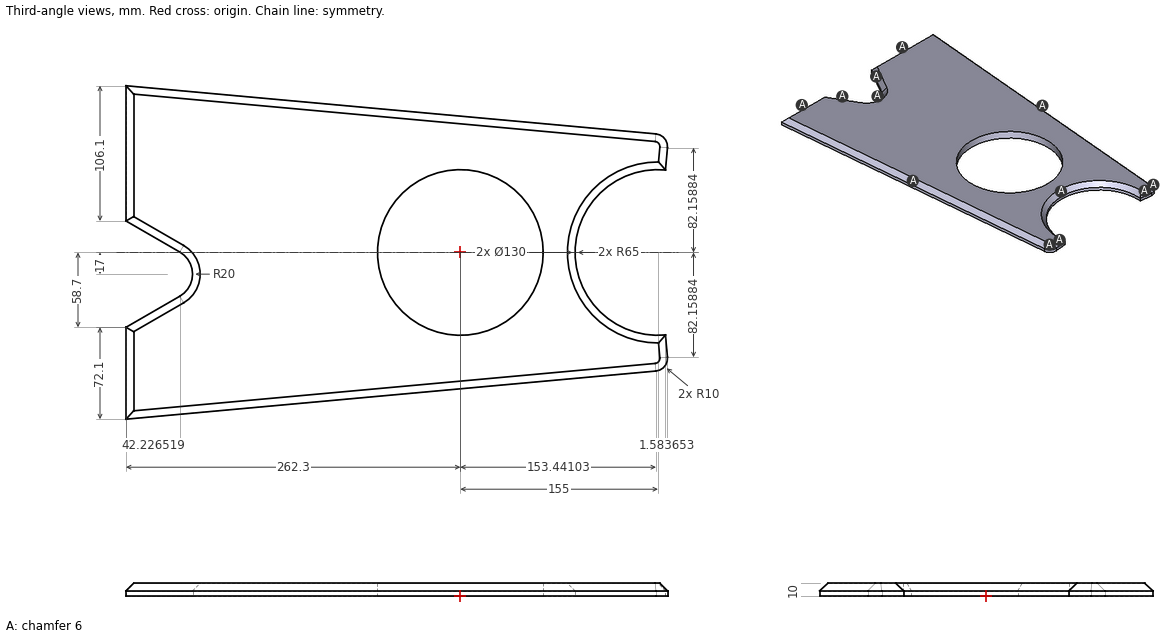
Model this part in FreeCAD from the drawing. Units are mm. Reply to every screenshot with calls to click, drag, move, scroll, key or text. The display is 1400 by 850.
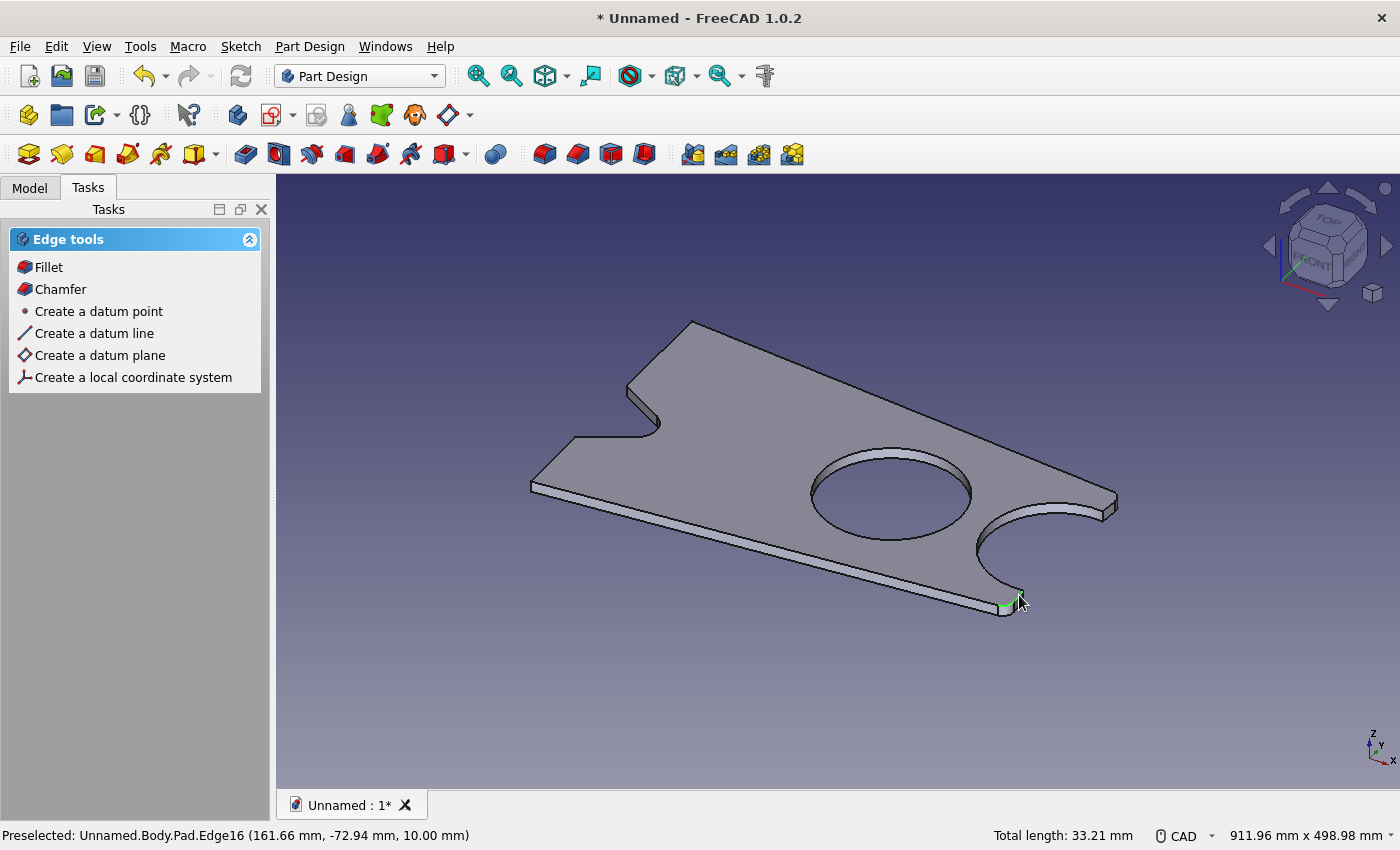
click(987, 525, ctrl)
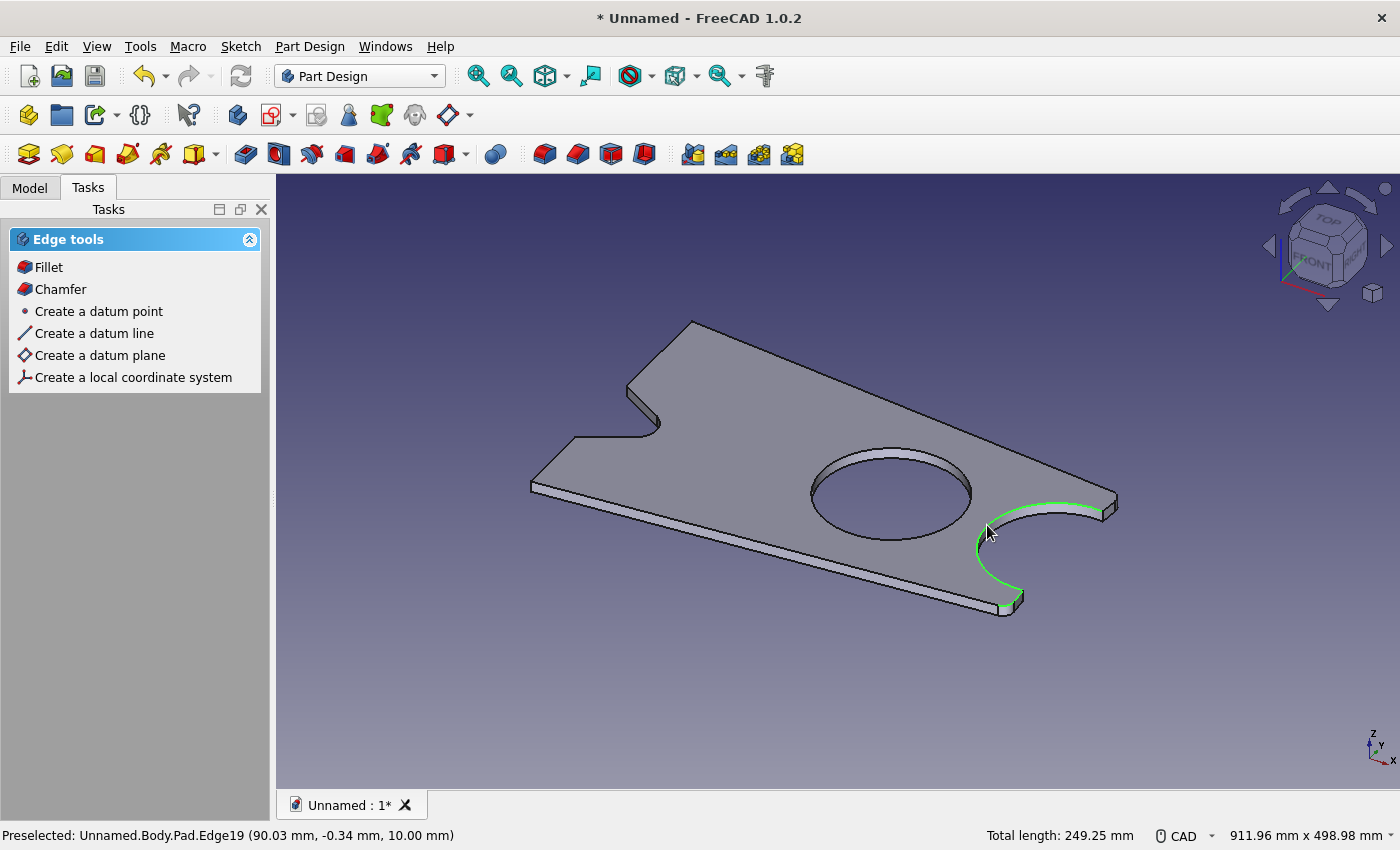
click(1109, 505, ctrl)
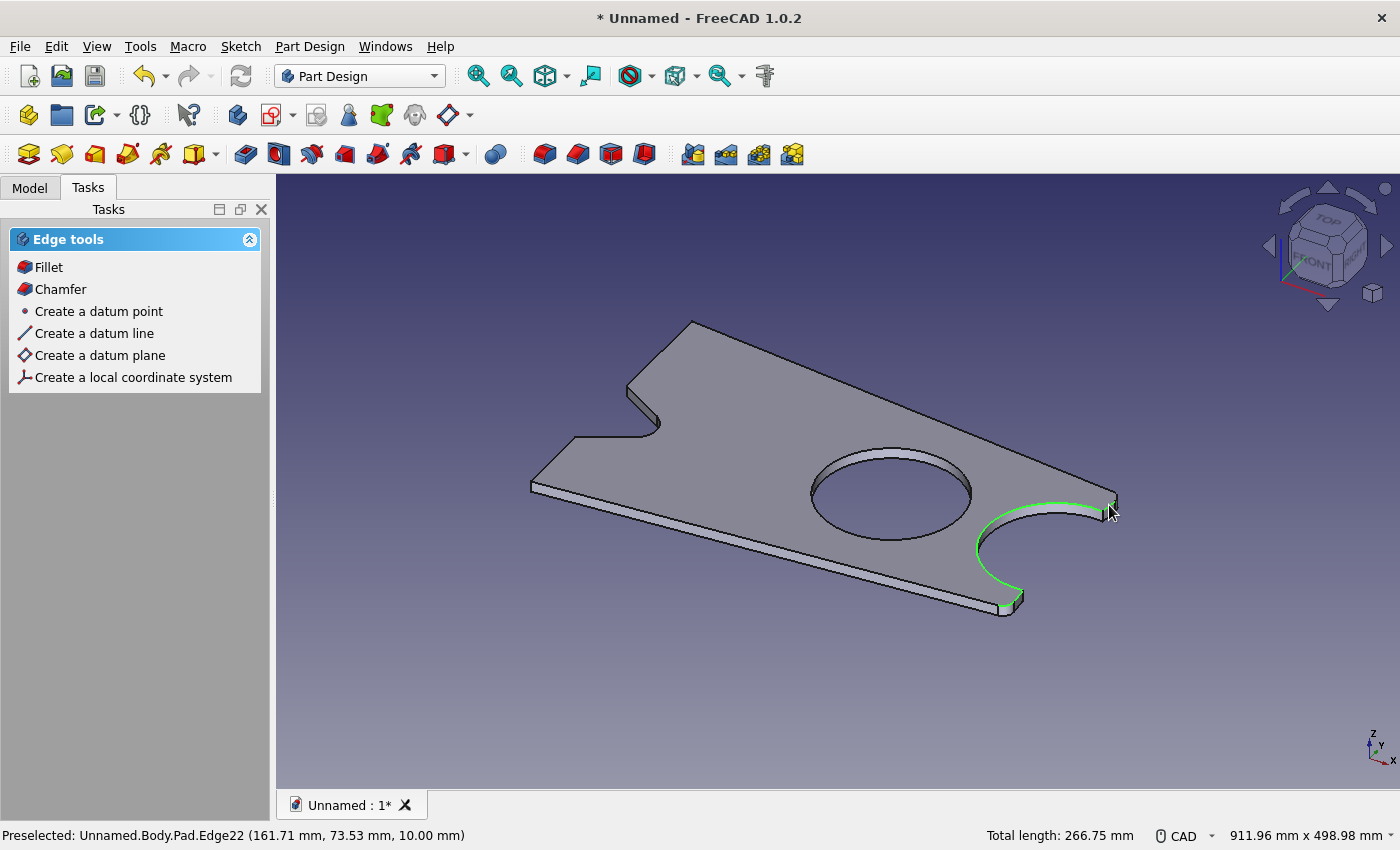
click(1117, 494, ctrl)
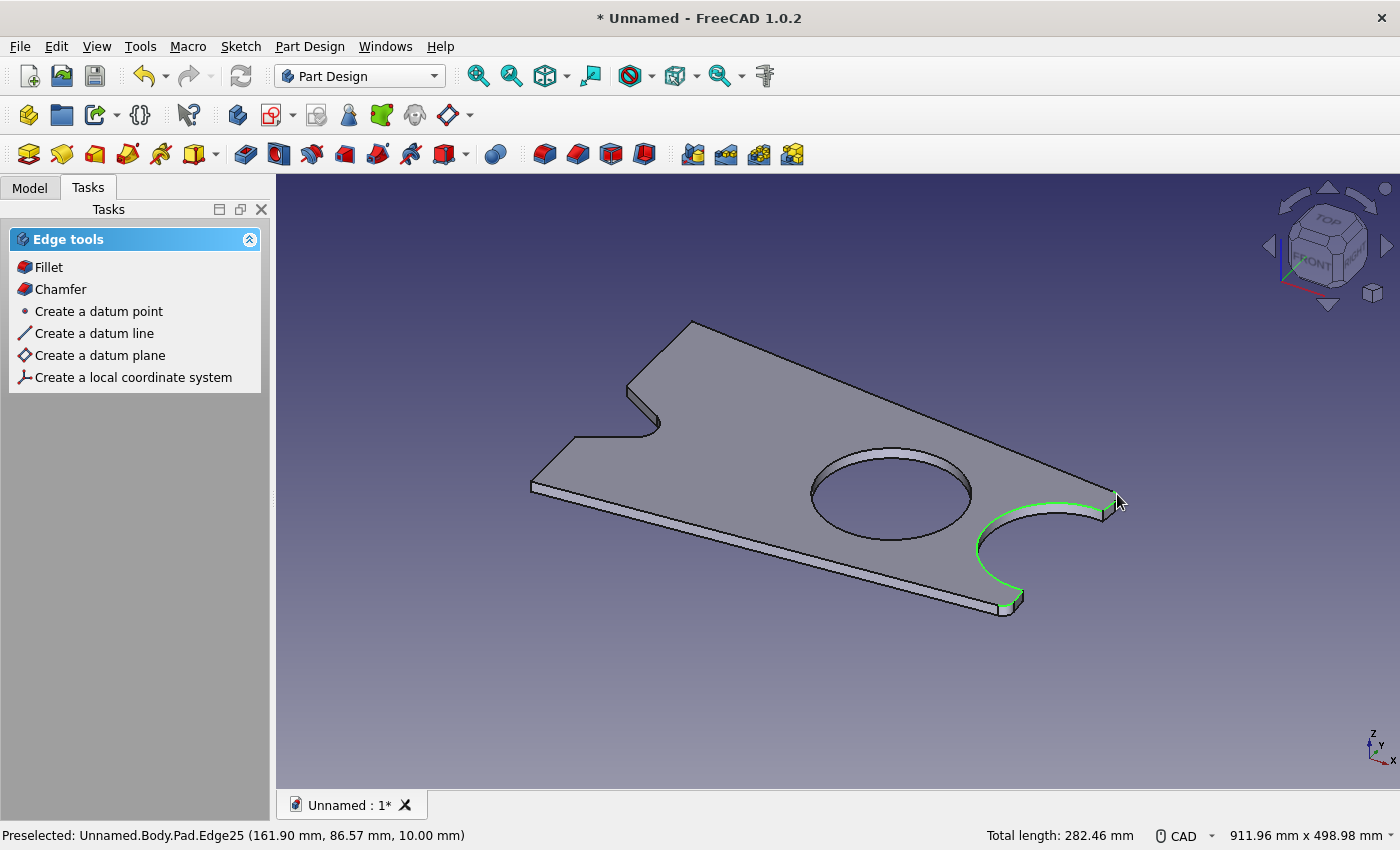
click(642, 400, ctrl)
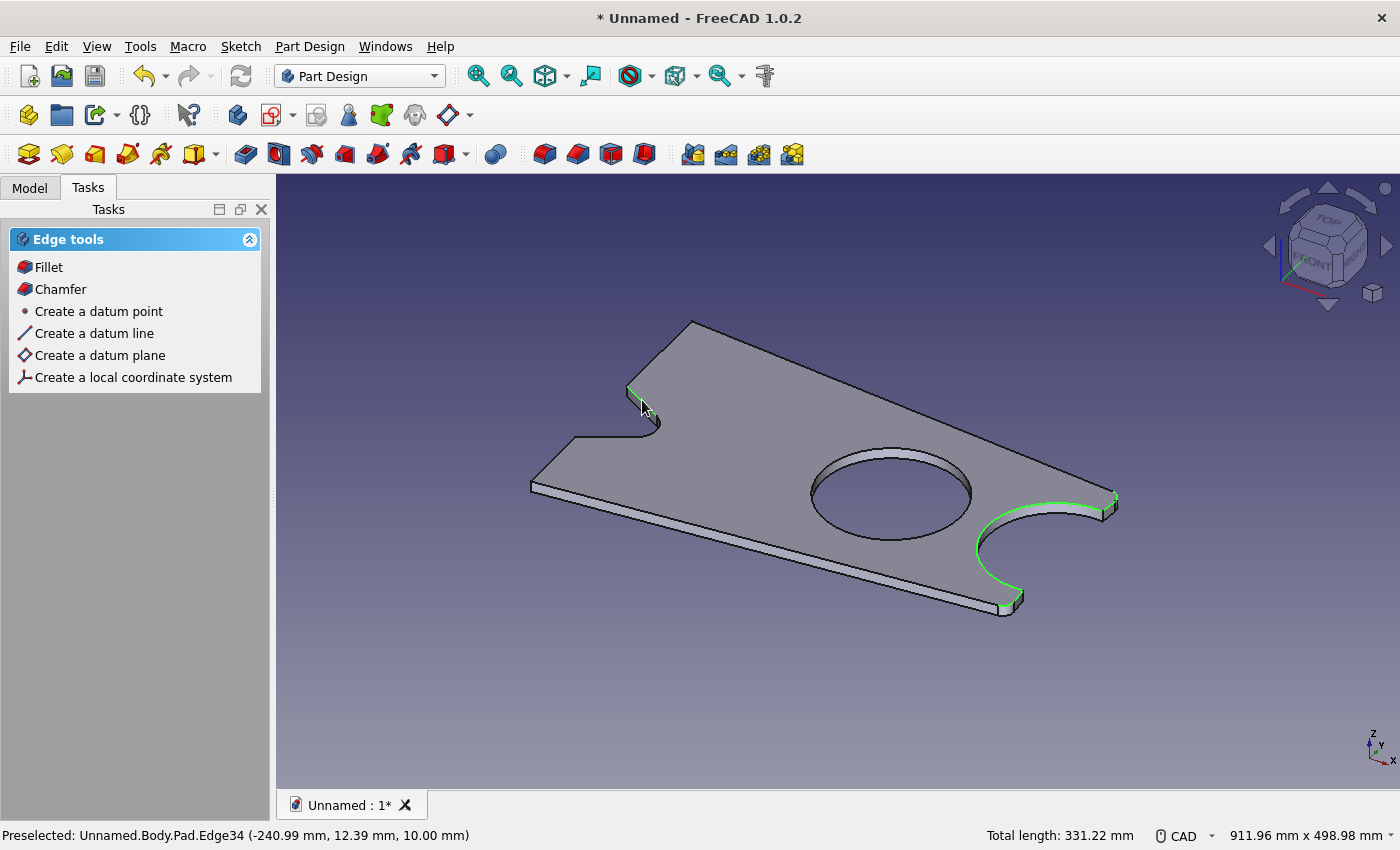
click(657, 429, ctrl)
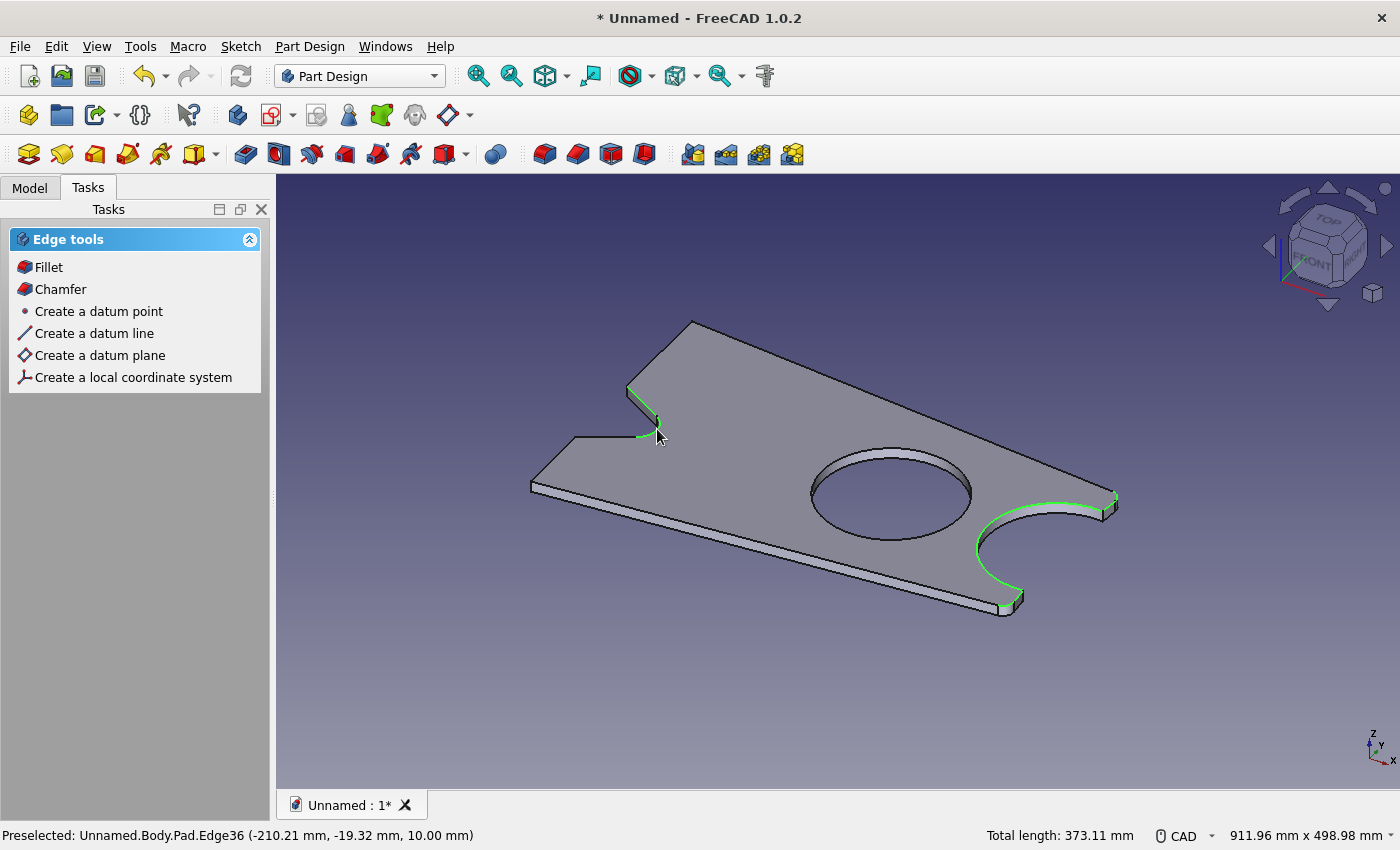
click(764, 542, ctrl)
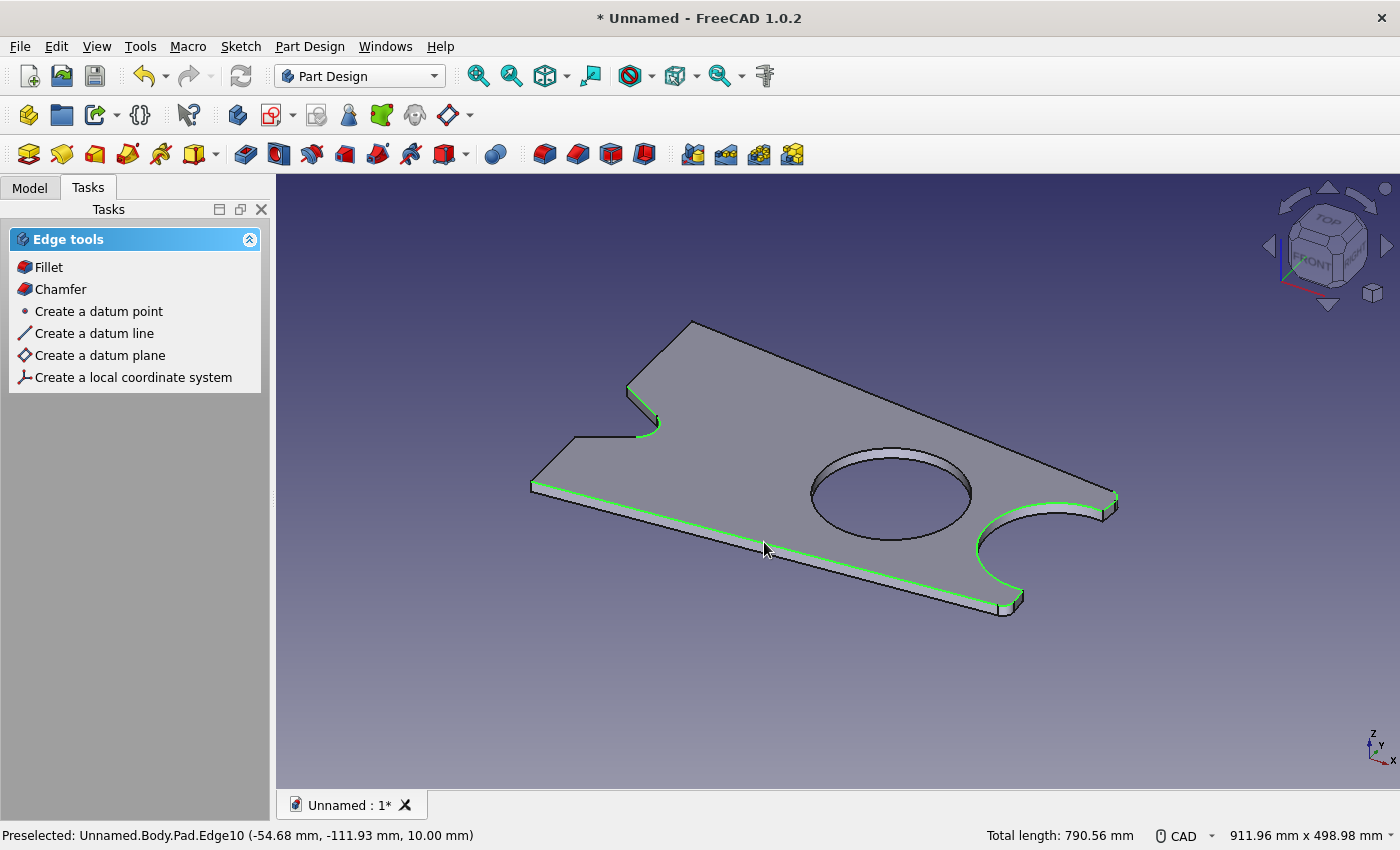
key(0)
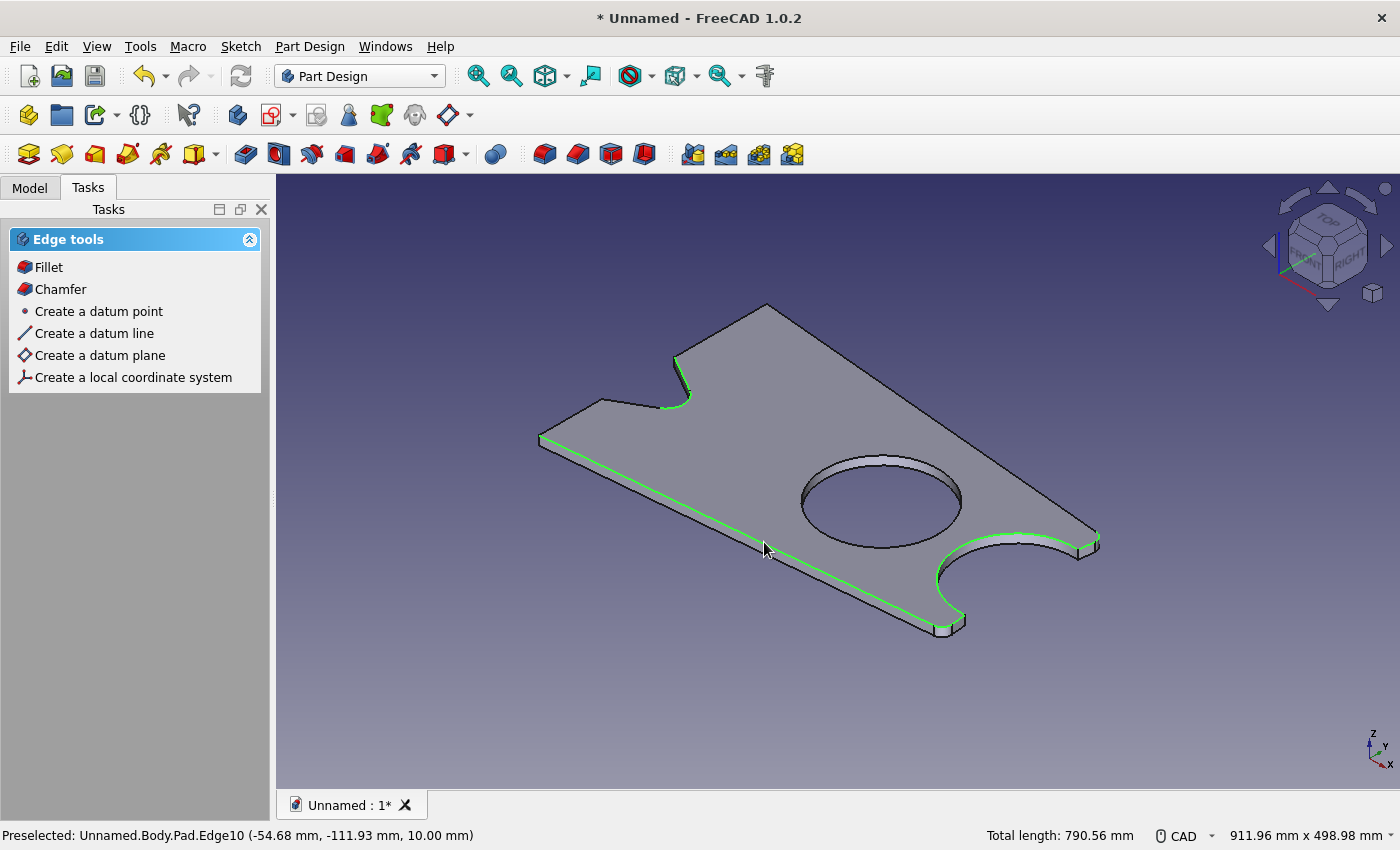
key(2)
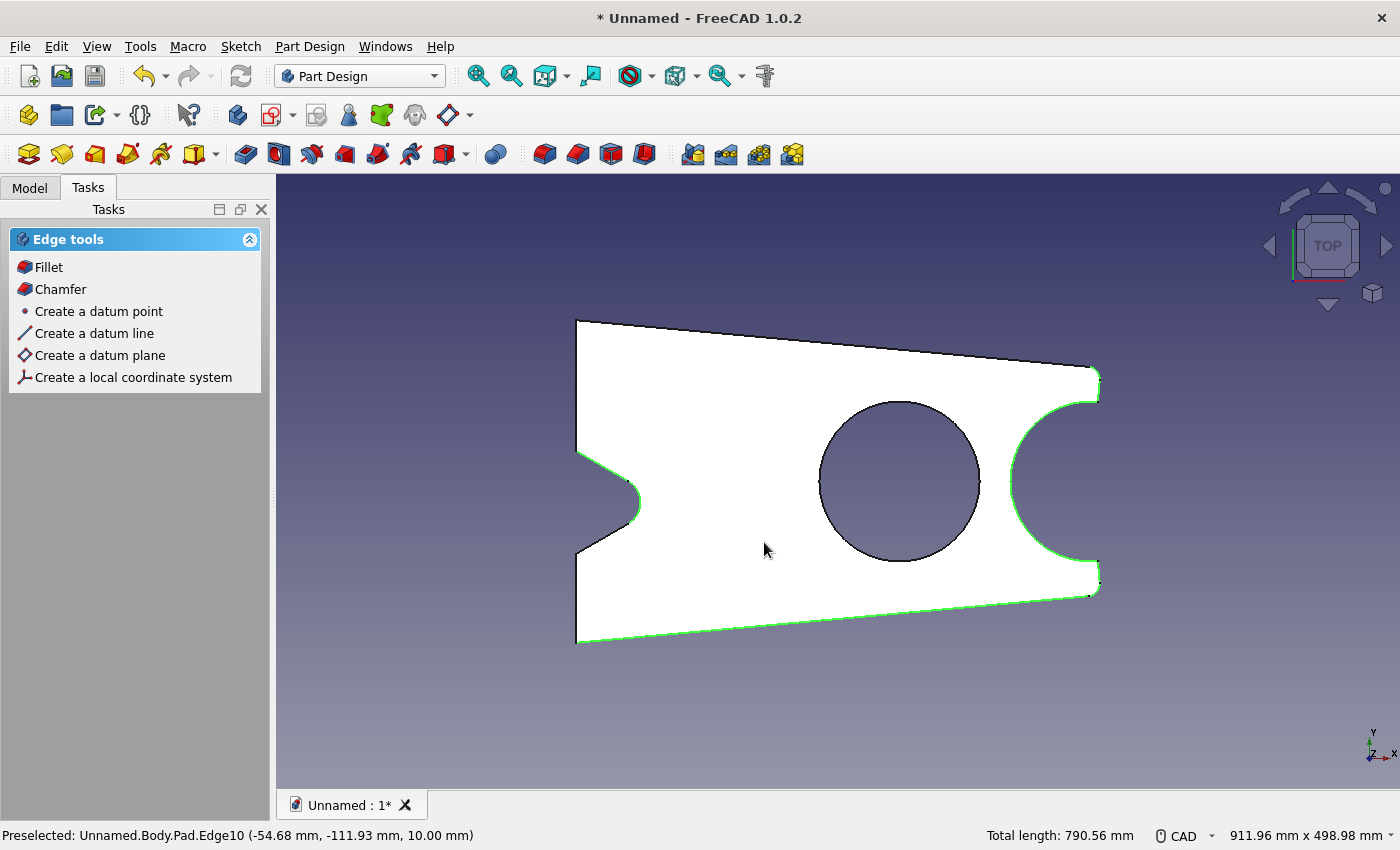
click(832, 343, ctrl)